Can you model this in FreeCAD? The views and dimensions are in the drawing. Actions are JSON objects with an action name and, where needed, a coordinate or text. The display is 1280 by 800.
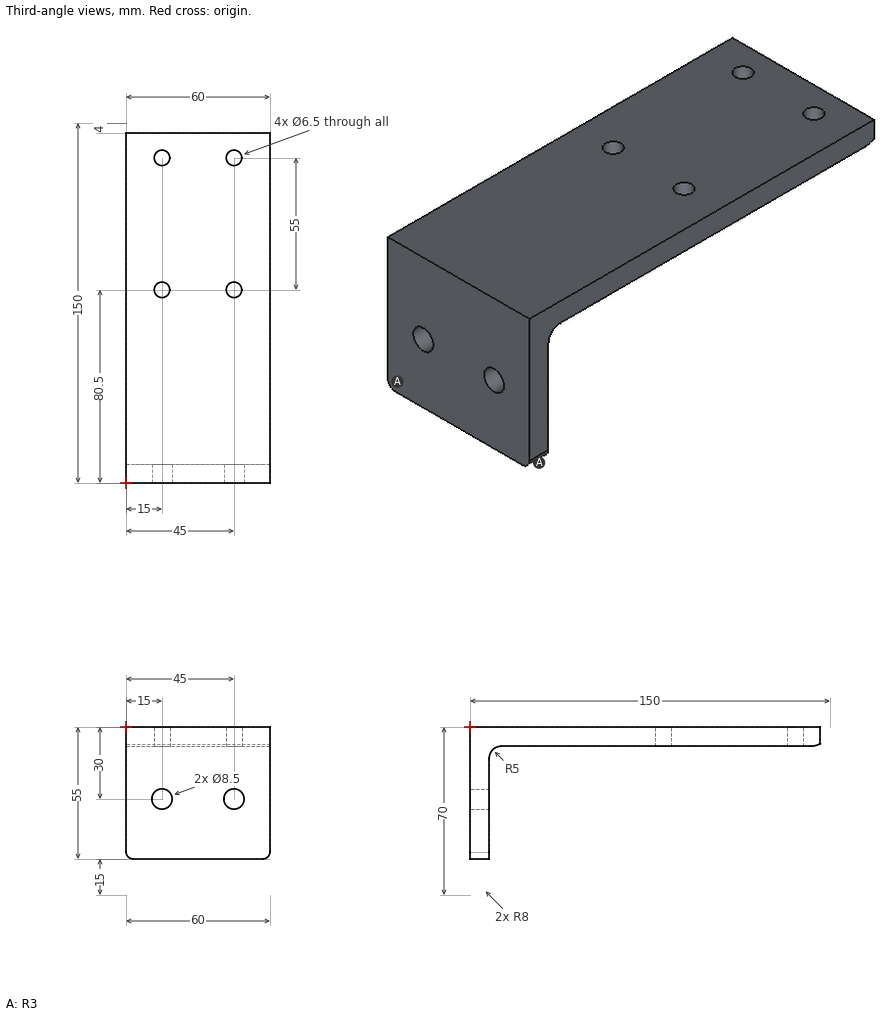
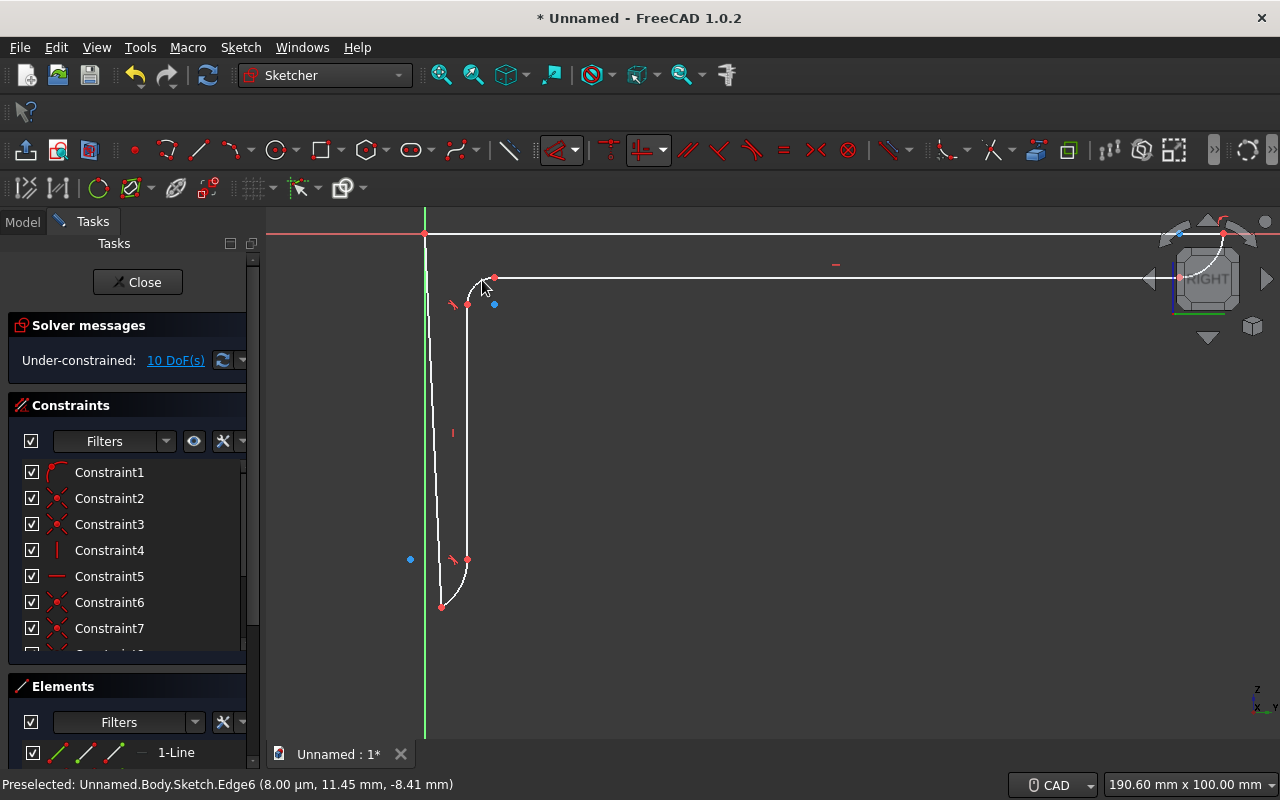
{"action": "left_click", "coordinate": [700, 278]}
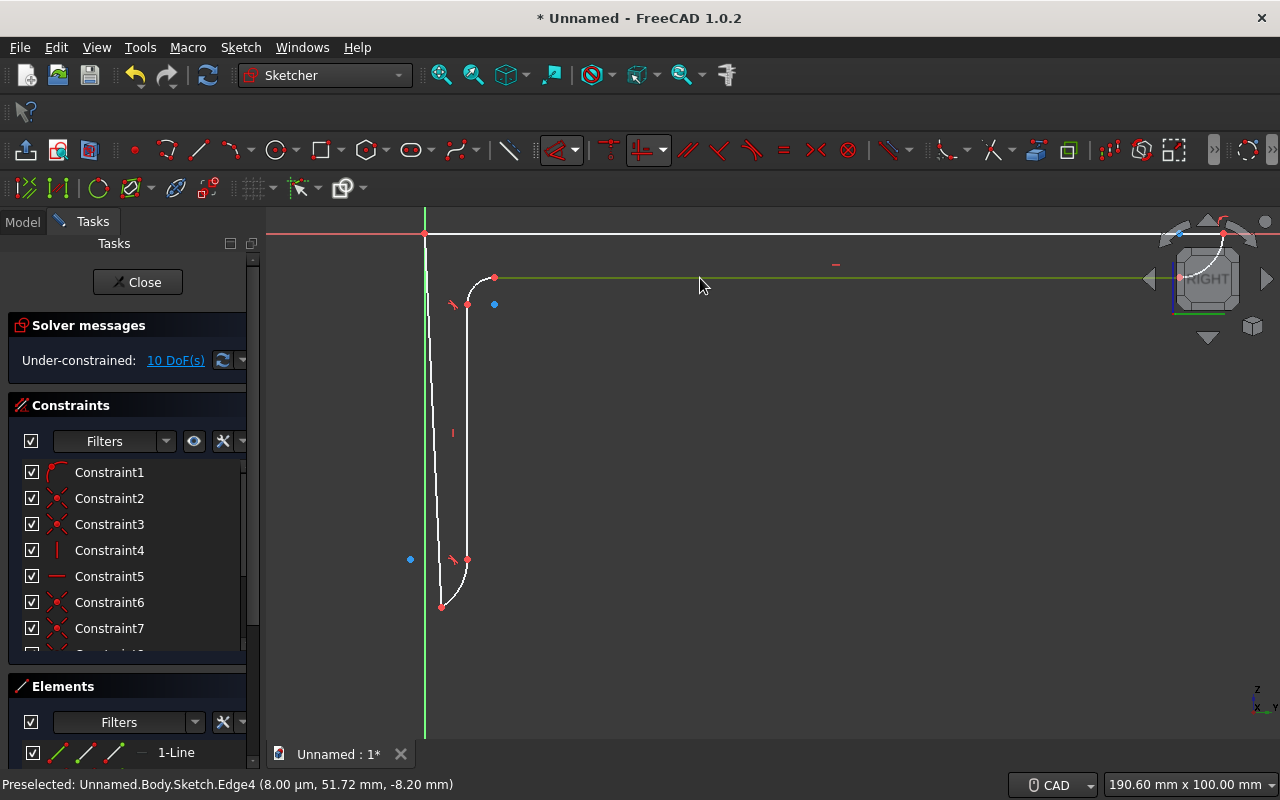
{"action": "left_click", "coordinate": [482, 281]}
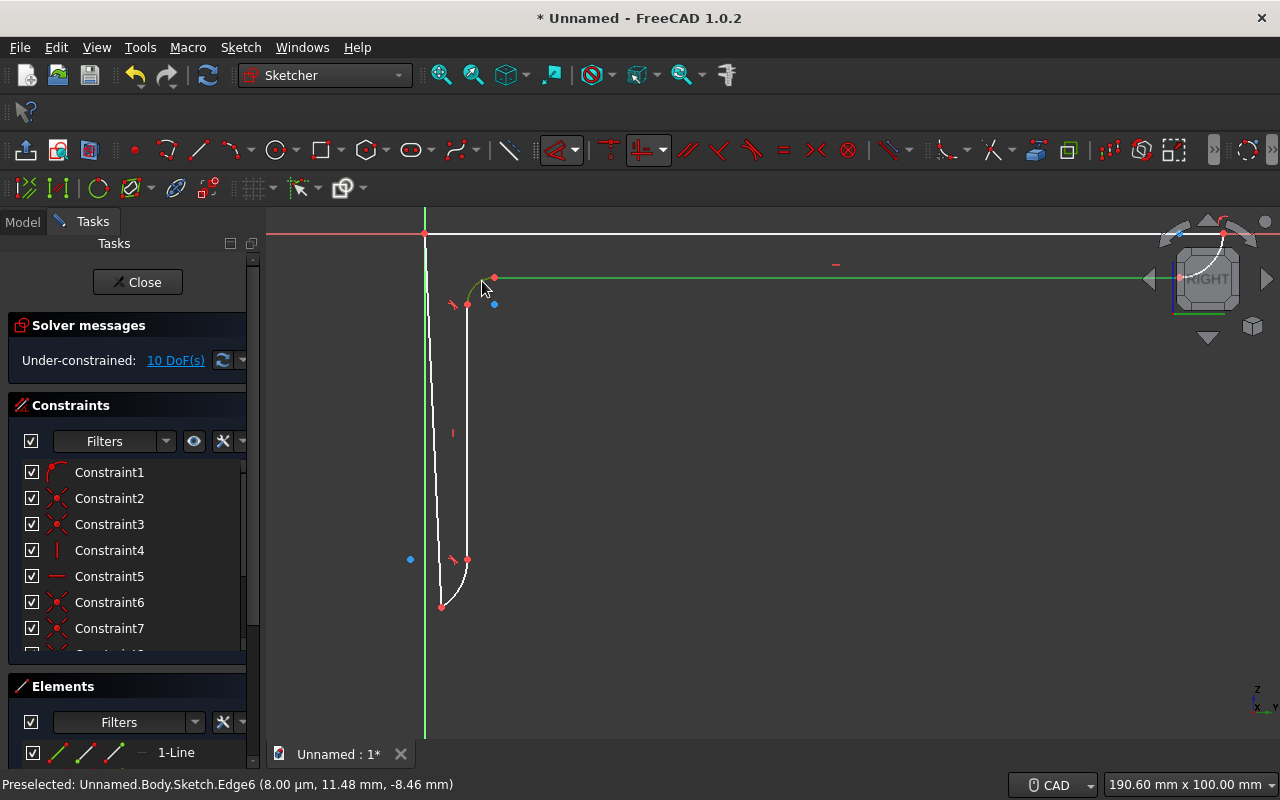
{"action": "key", "text": "t"}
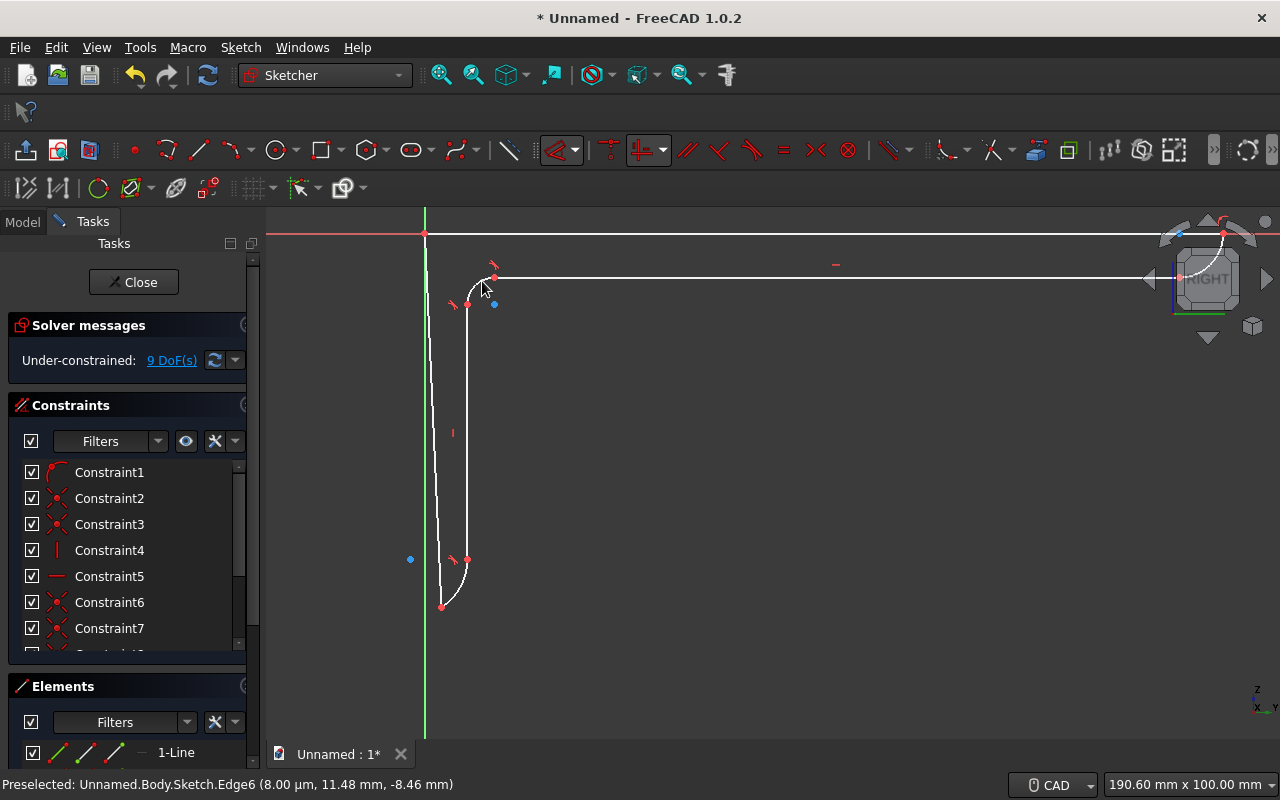
{"action": "left_click", "coordinate": [700, 278]}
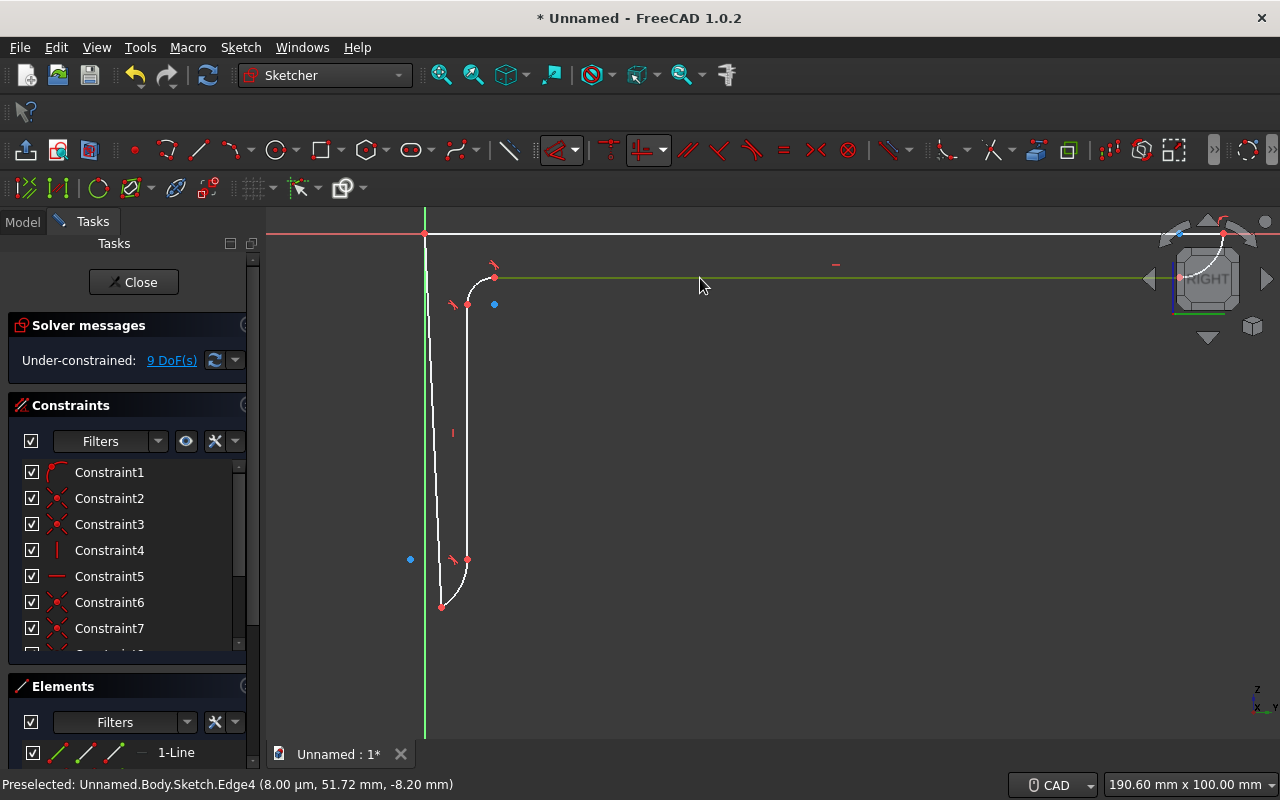
{"action": "scroll", "coordinate": [462, 580], "scroll_direction": "down", "scroll_amount": 2}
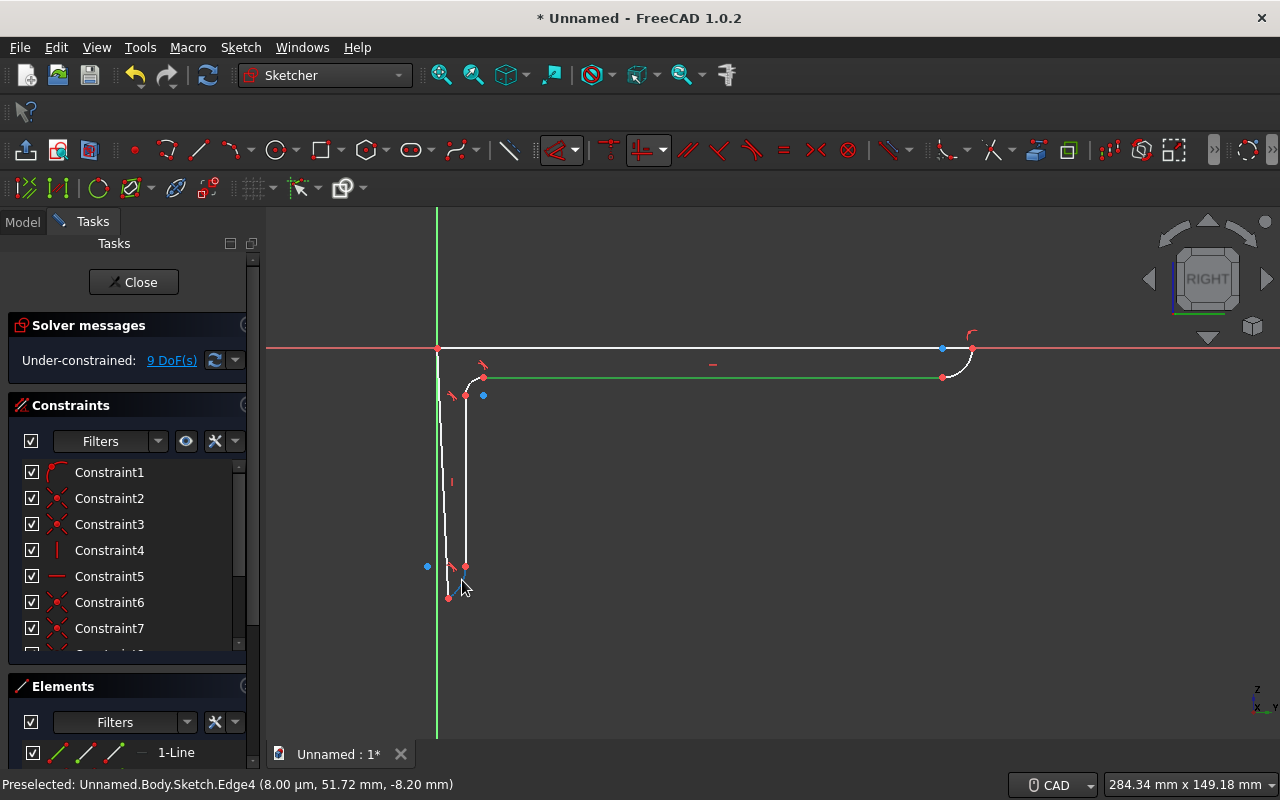
{"action": "left_click", "coordinate": [956, 374]}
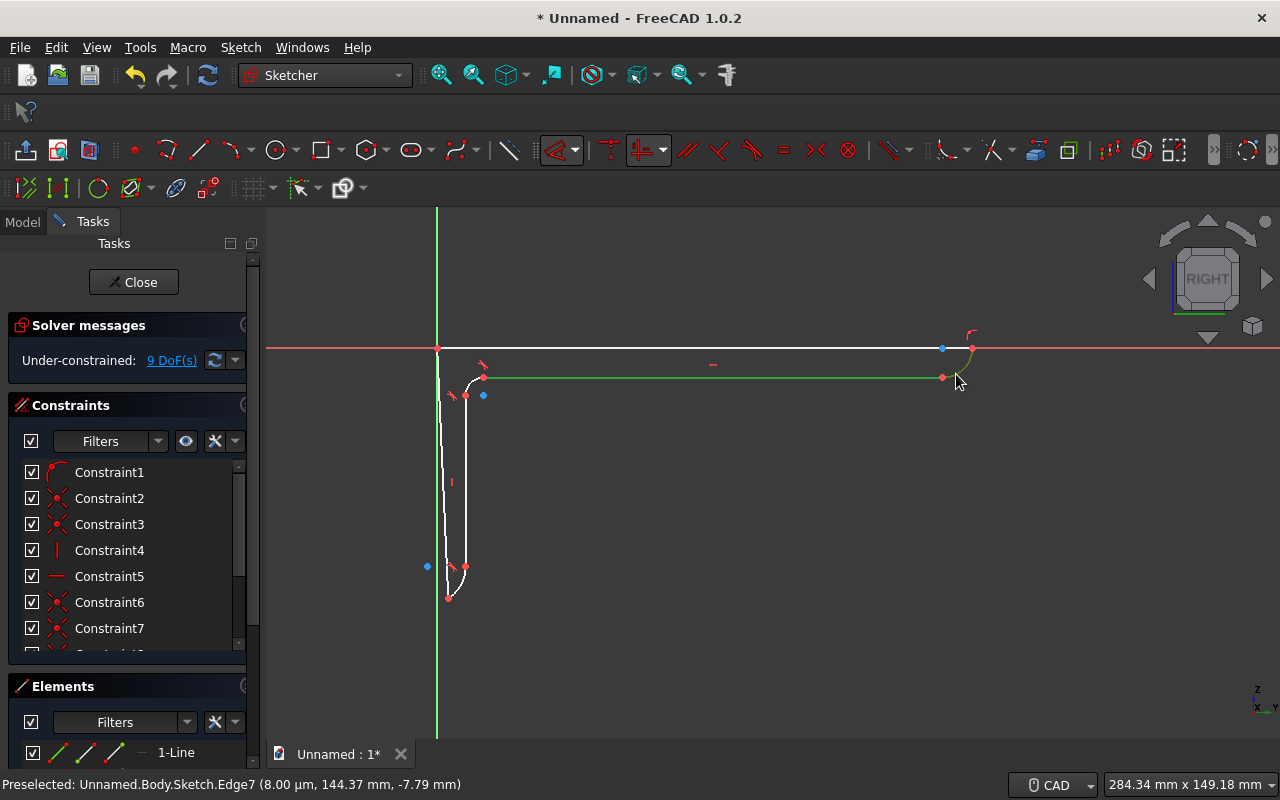
{"action": "key", "text": "t"}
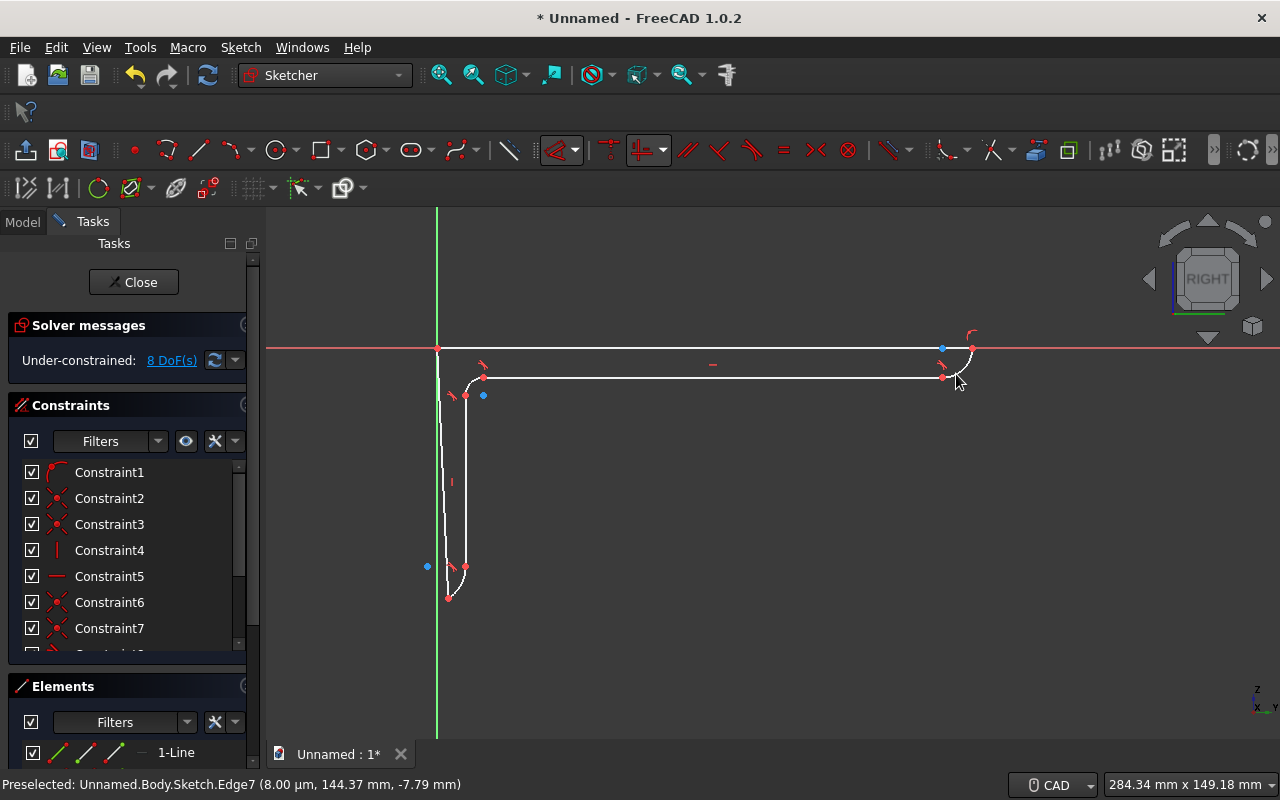
{"action": "left_click", "coordinate": [441, 423]}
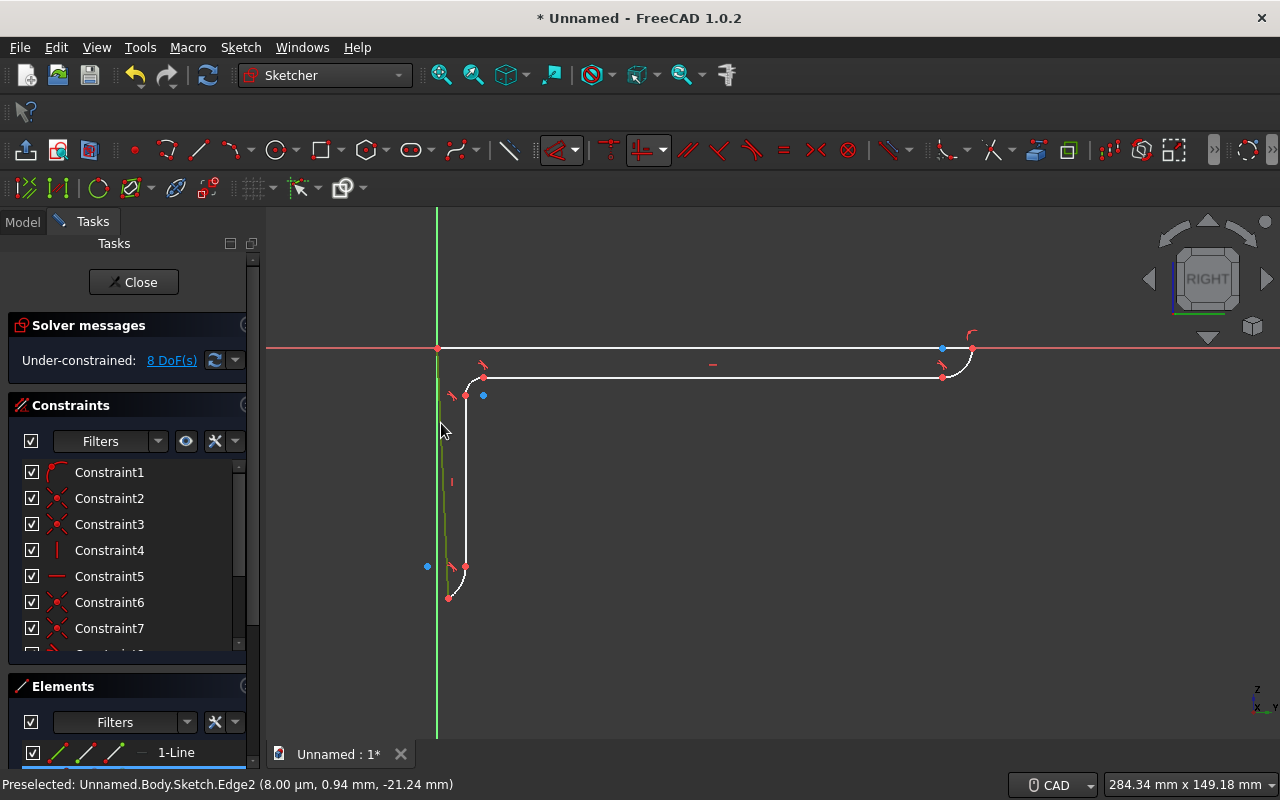
{"action": "left_click", "coordinate": [666, 150]}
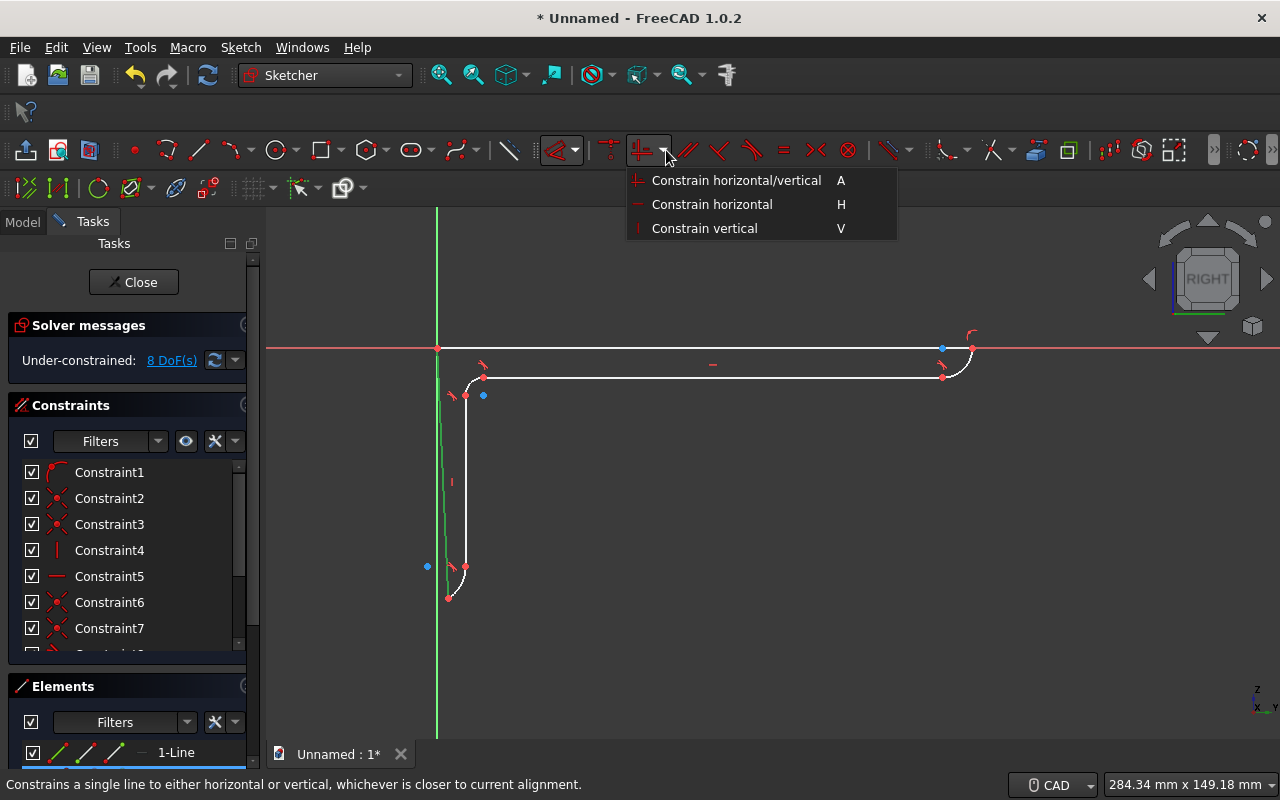
{"action": "left_click", "coordinate": [762, 228]}